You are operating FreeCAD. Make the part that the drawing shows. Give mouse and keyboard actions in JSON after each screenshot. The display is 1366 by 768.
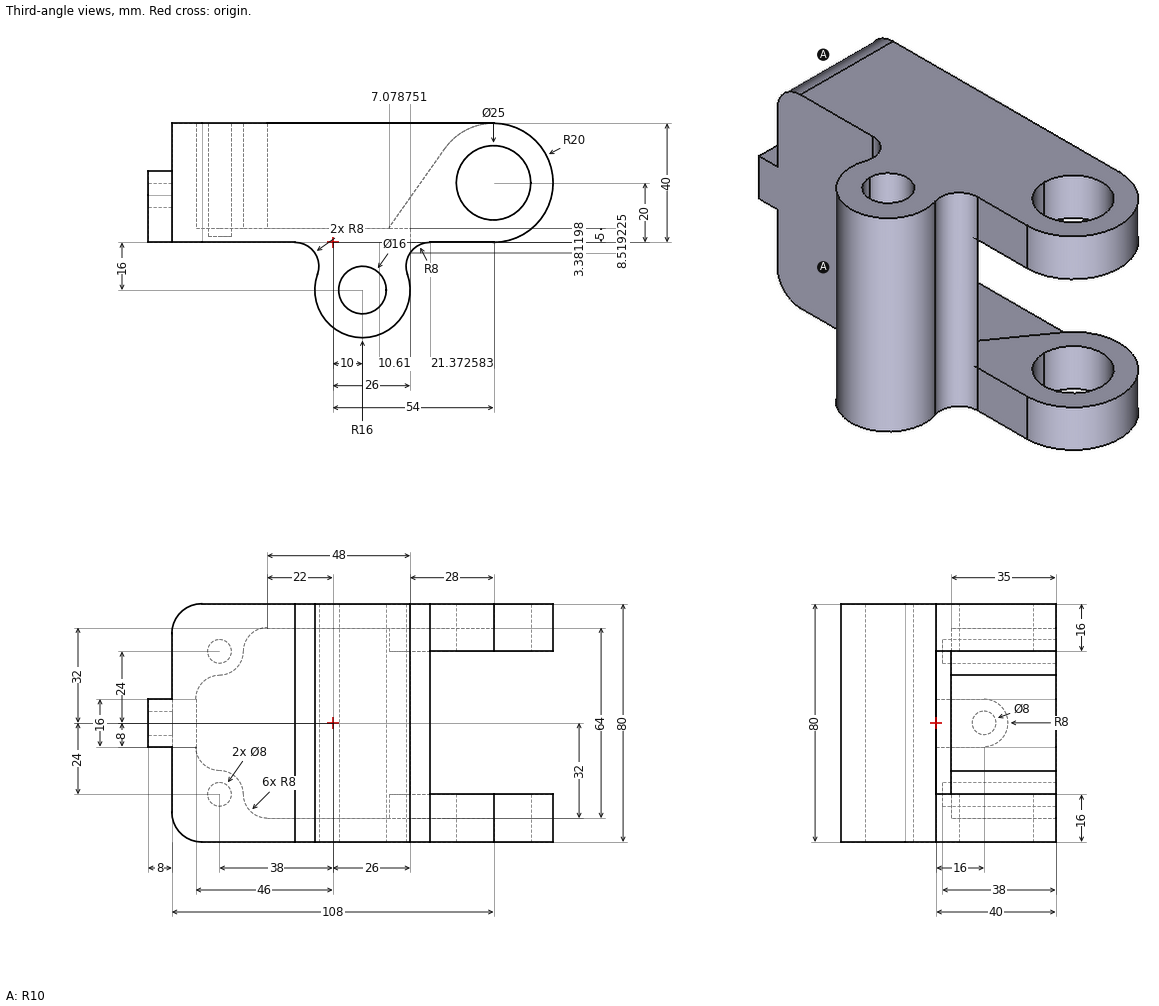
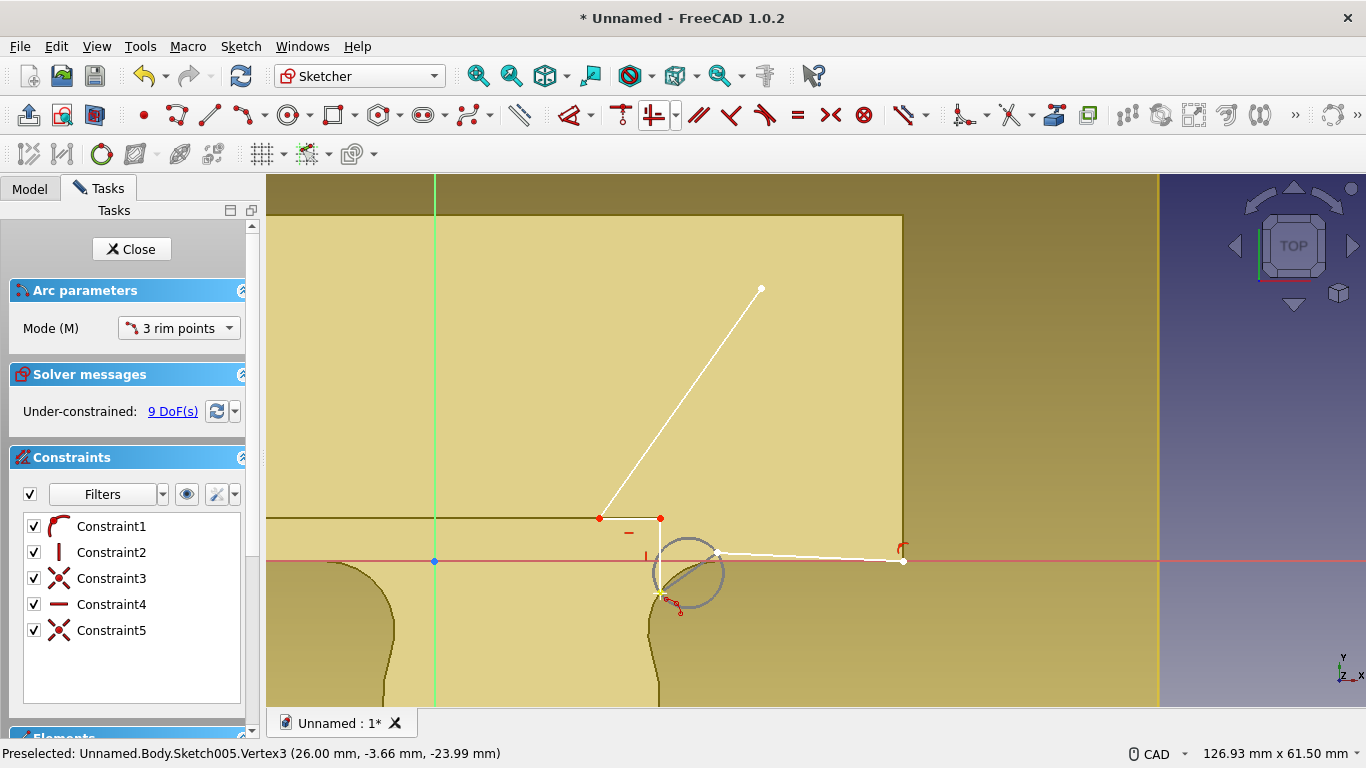
{"action": "scroll", "coordinate": [685, 569], "scroll_direction": "up", "scroll_amount": 4}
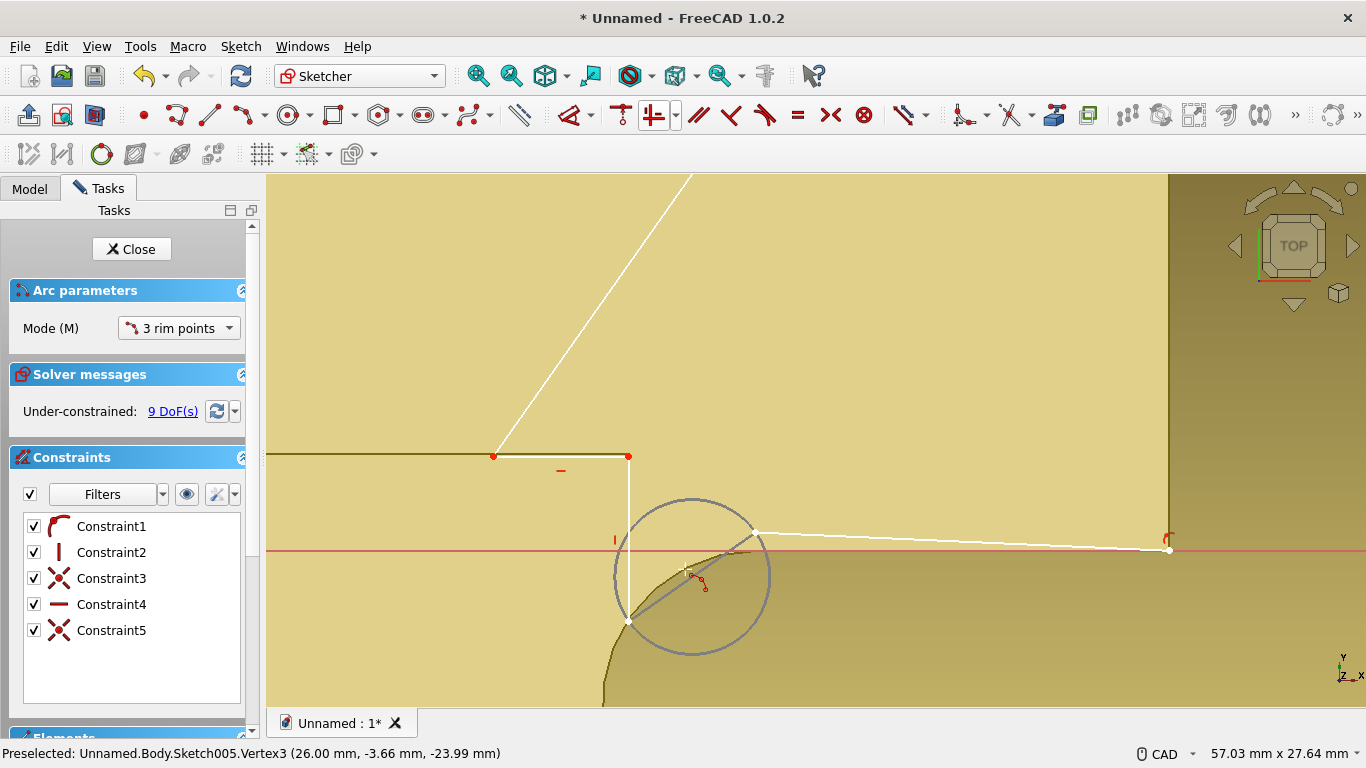
{"action": "left_click", "coordinate": [684, 569]}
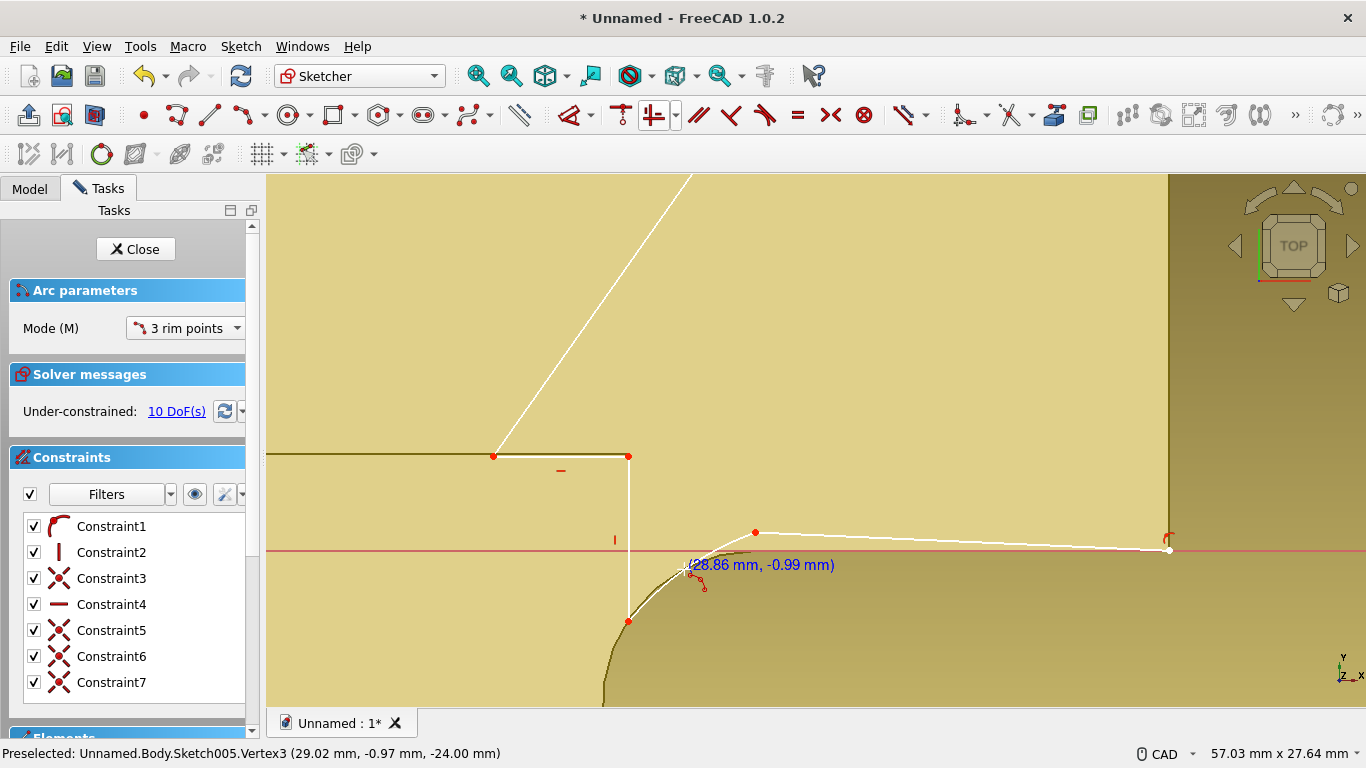
{"action": "scroll", "coordinate": [689, 571], "scroll_direction": "down", "scroll_amount": 4}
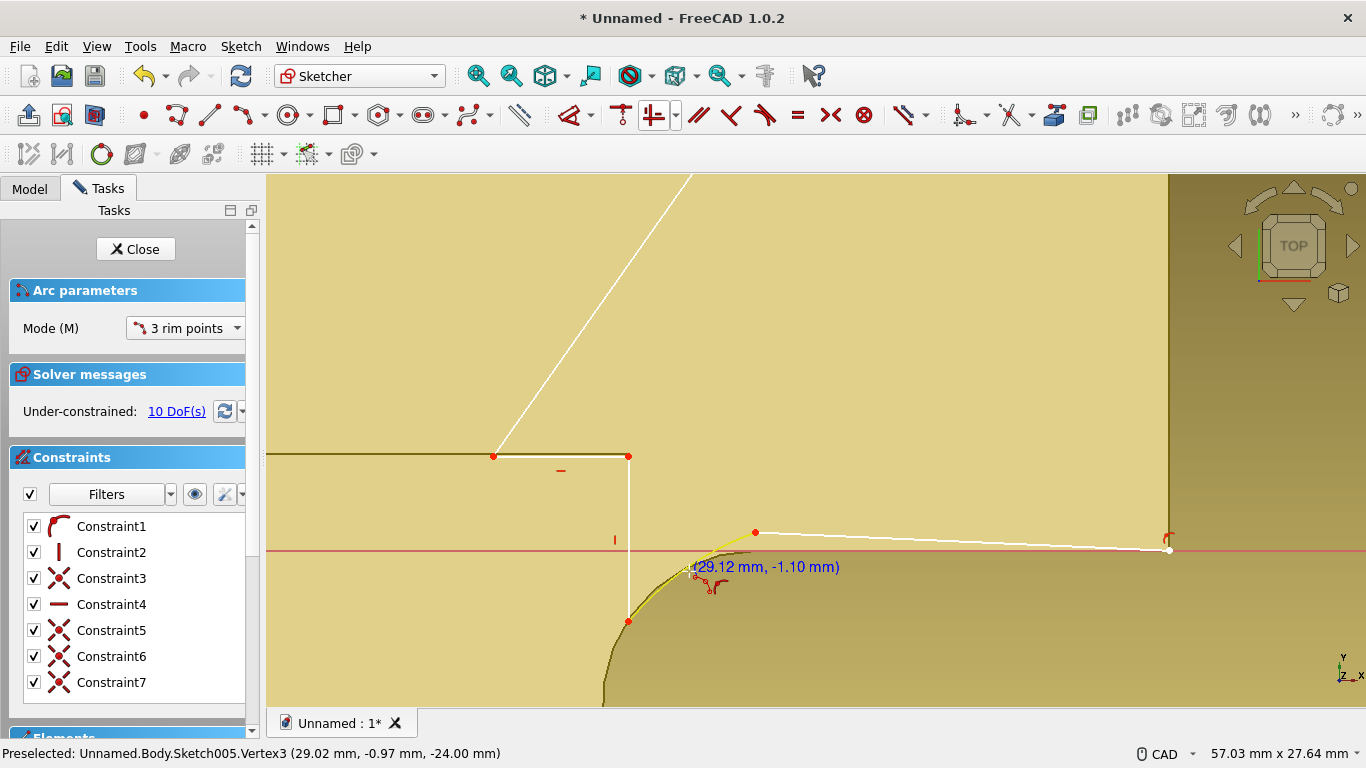
{"action": "left_click", "coordinate": [763, 290]}
{"action": "left_click", "coordinate": [905, 562]}
{"action": "left_click", "coordinate": [1059, 309]}
{"action": "key", "text": "Escape"}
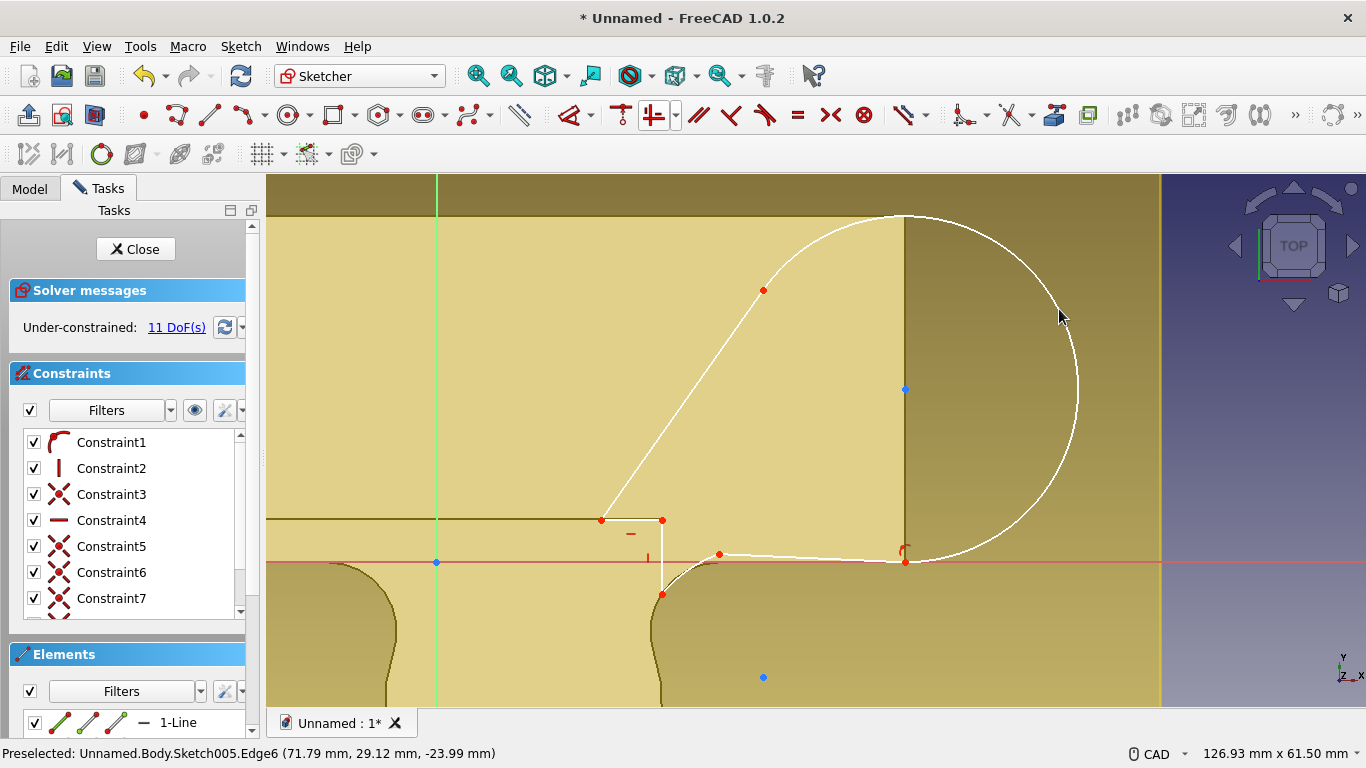
{"action": "left_click", "coordinate": [849, 560]}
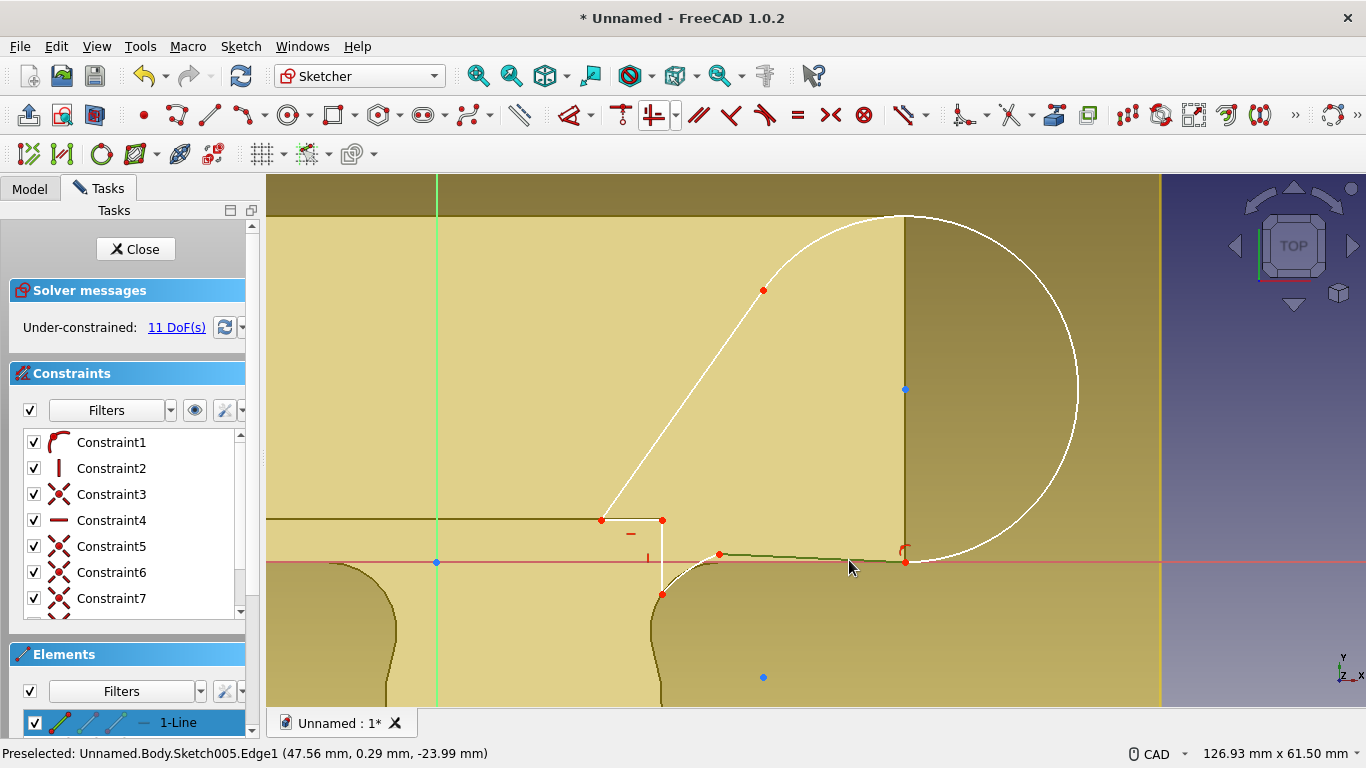
{"action": "left_click", "coordinate": [700, 563]}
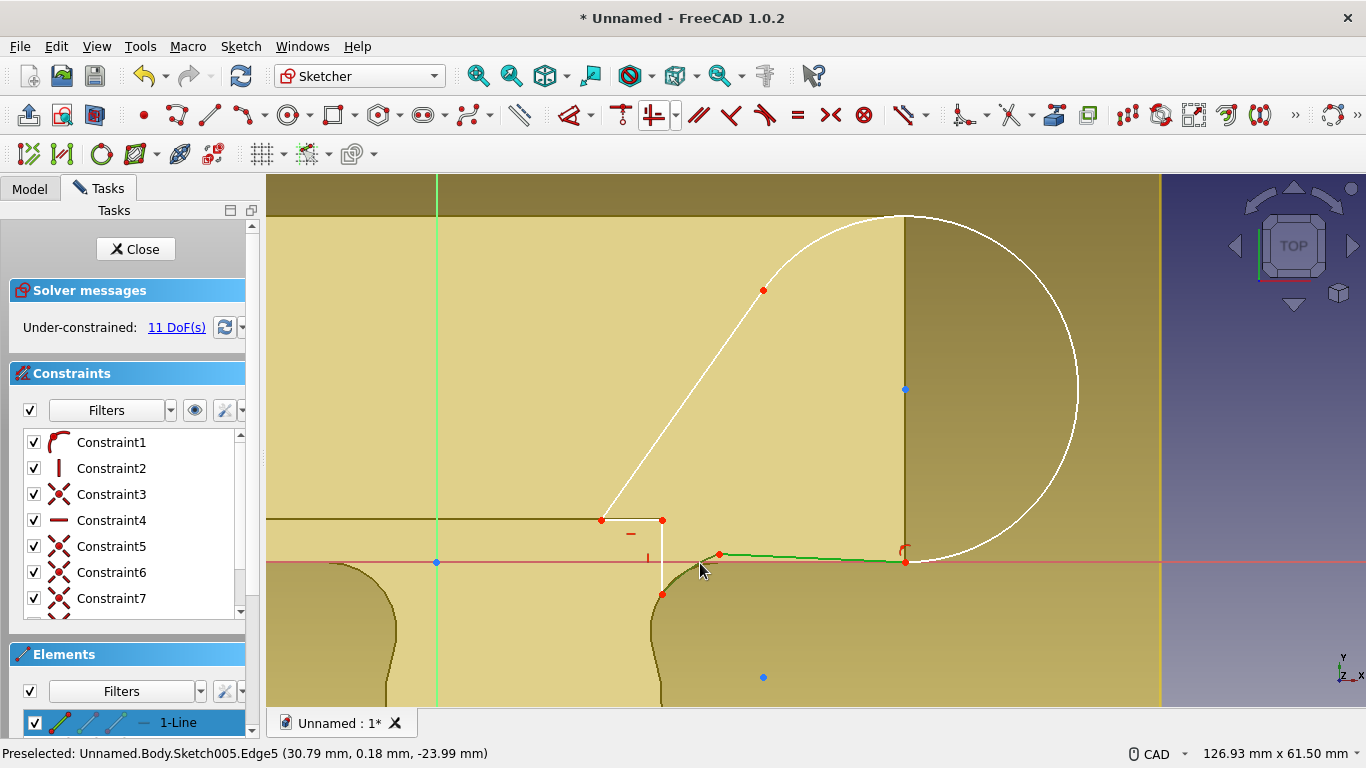
{"action": "key", "text": "t"}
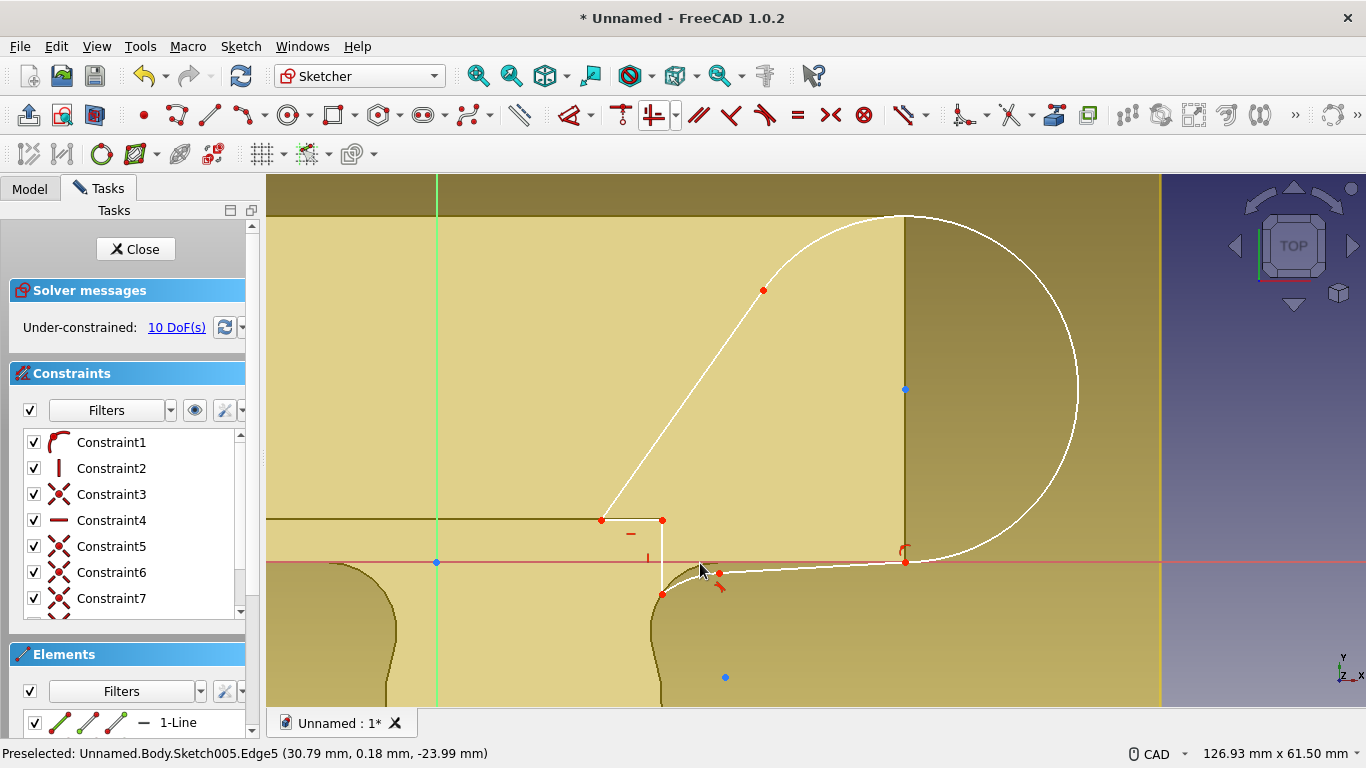
{"action": "left_click", "coordinate": [849, 566]}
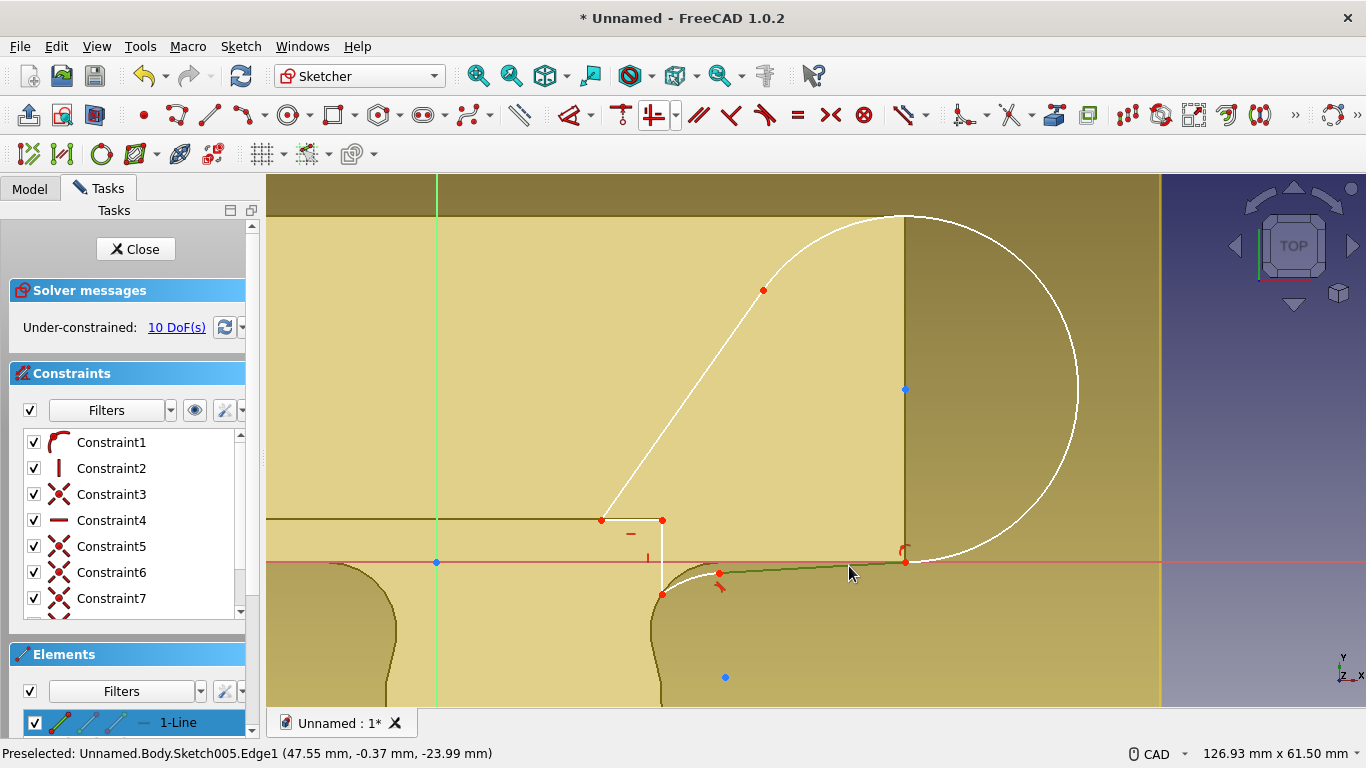
{"action": "left_click", "coordinate": [1068, 447]}